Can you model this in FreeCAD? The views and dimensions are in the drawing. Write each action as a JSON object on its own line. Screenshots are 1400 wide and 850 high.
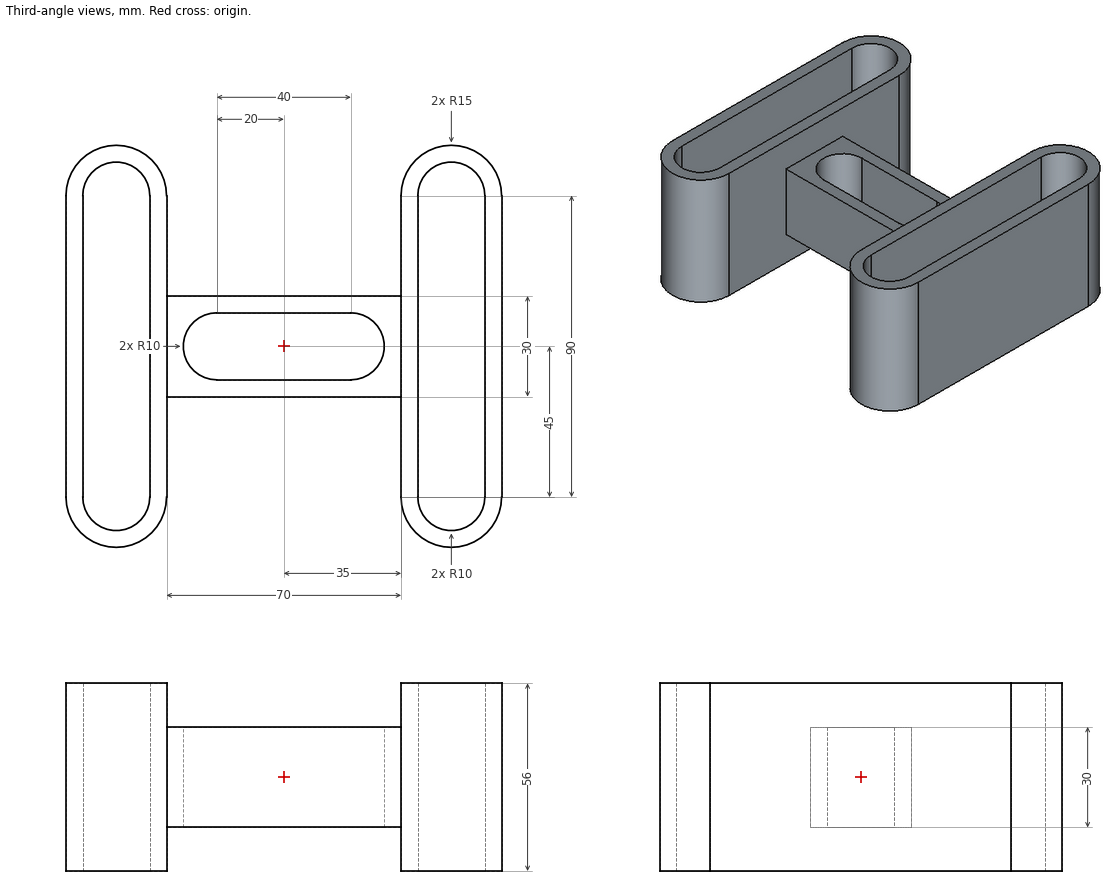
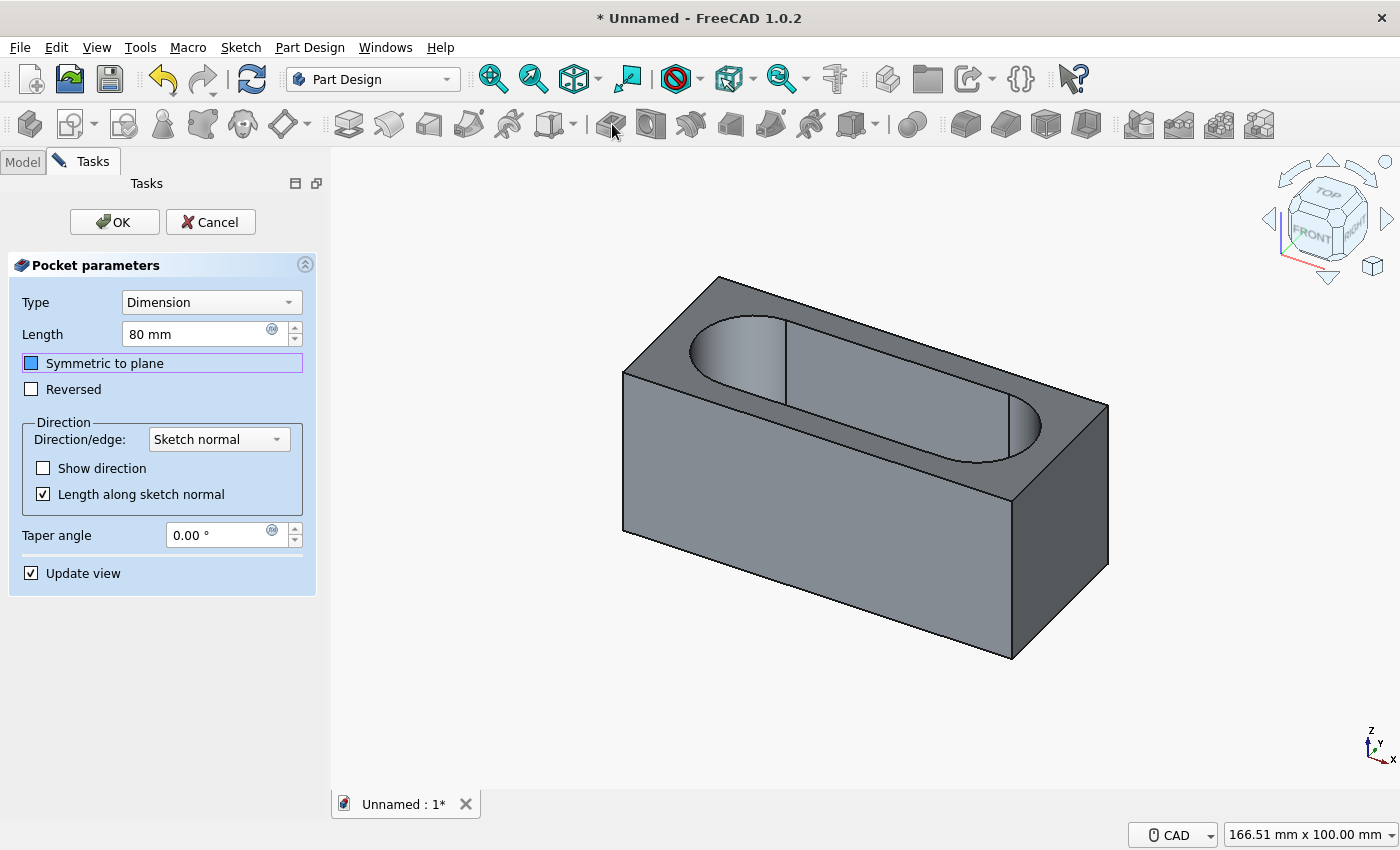
{"action": "left_click", "coordinate": [115, 222]}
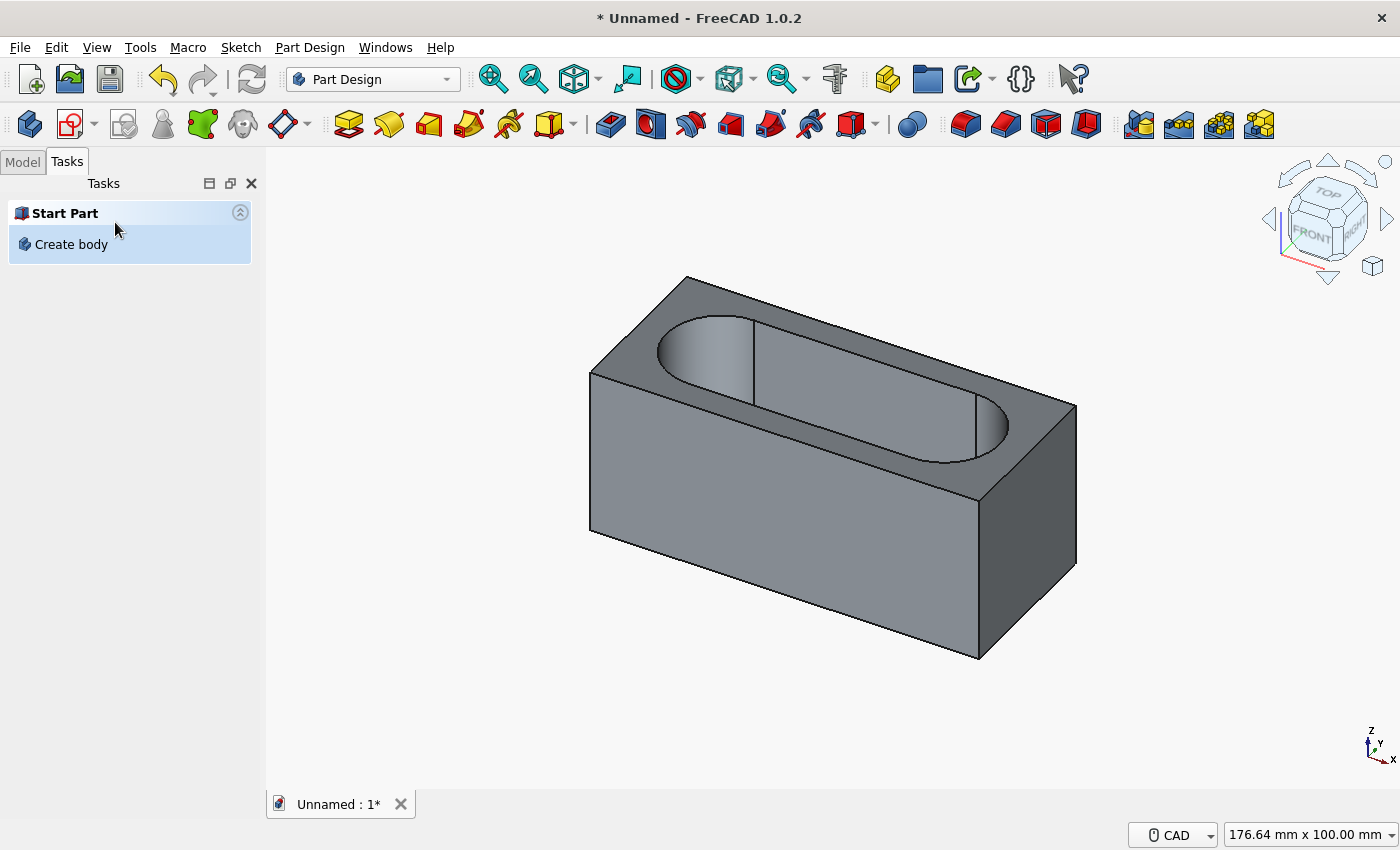
{"action": "left_click", "coordinate": [70, 124]}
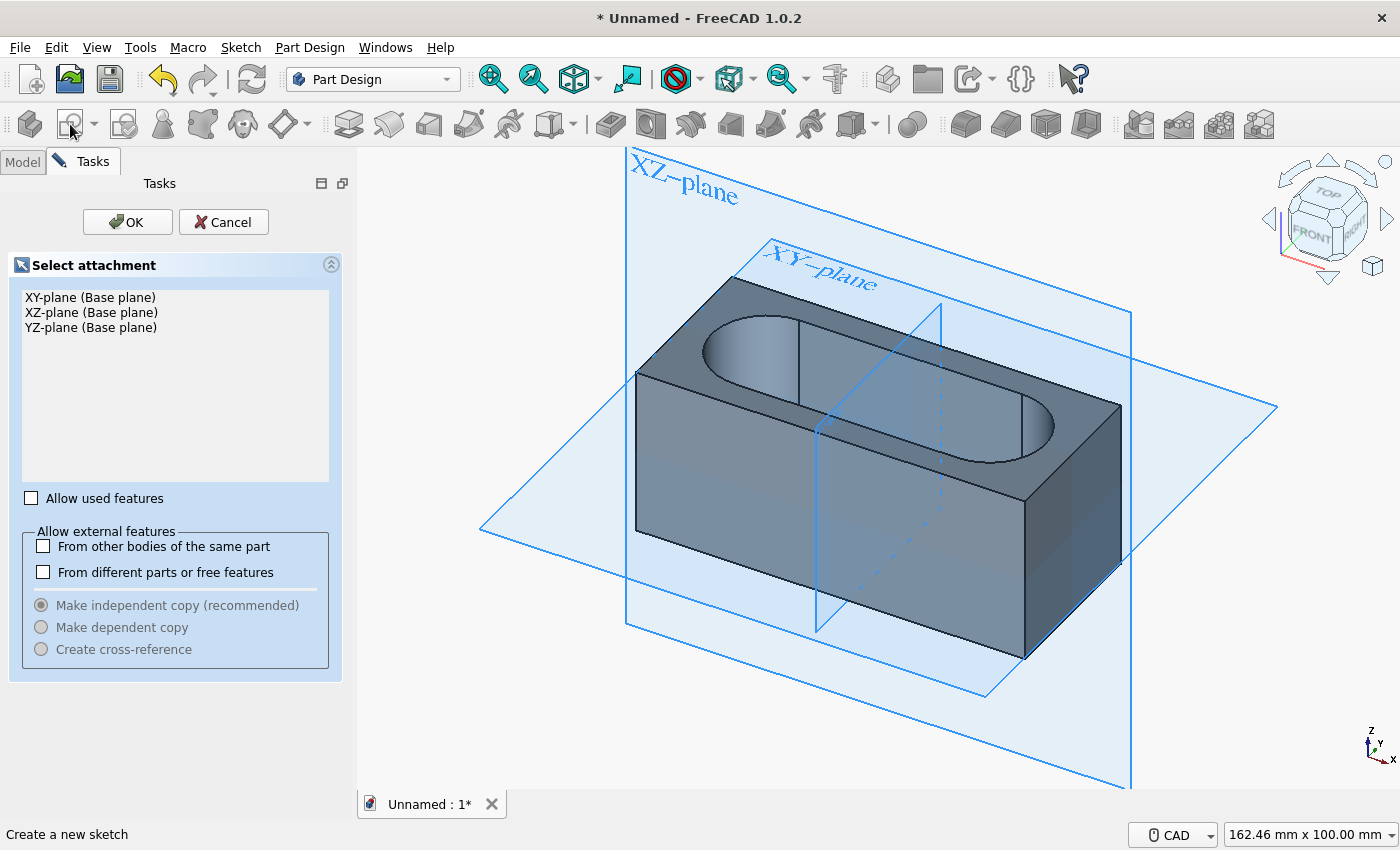
{"action": "left_click", "coordinate": [82, 298]}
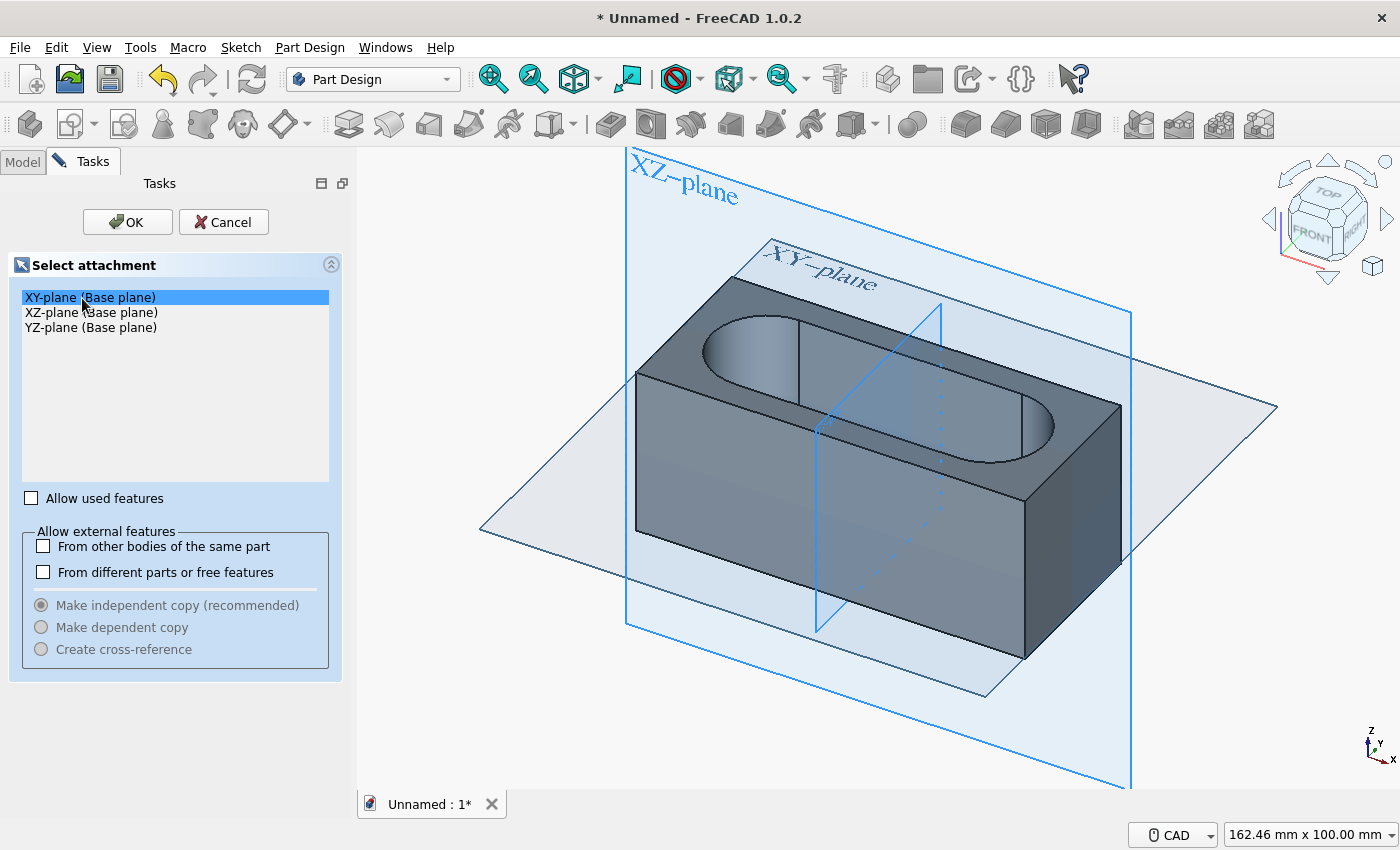
{"action": "left_click", "coordinate": [128, 222]}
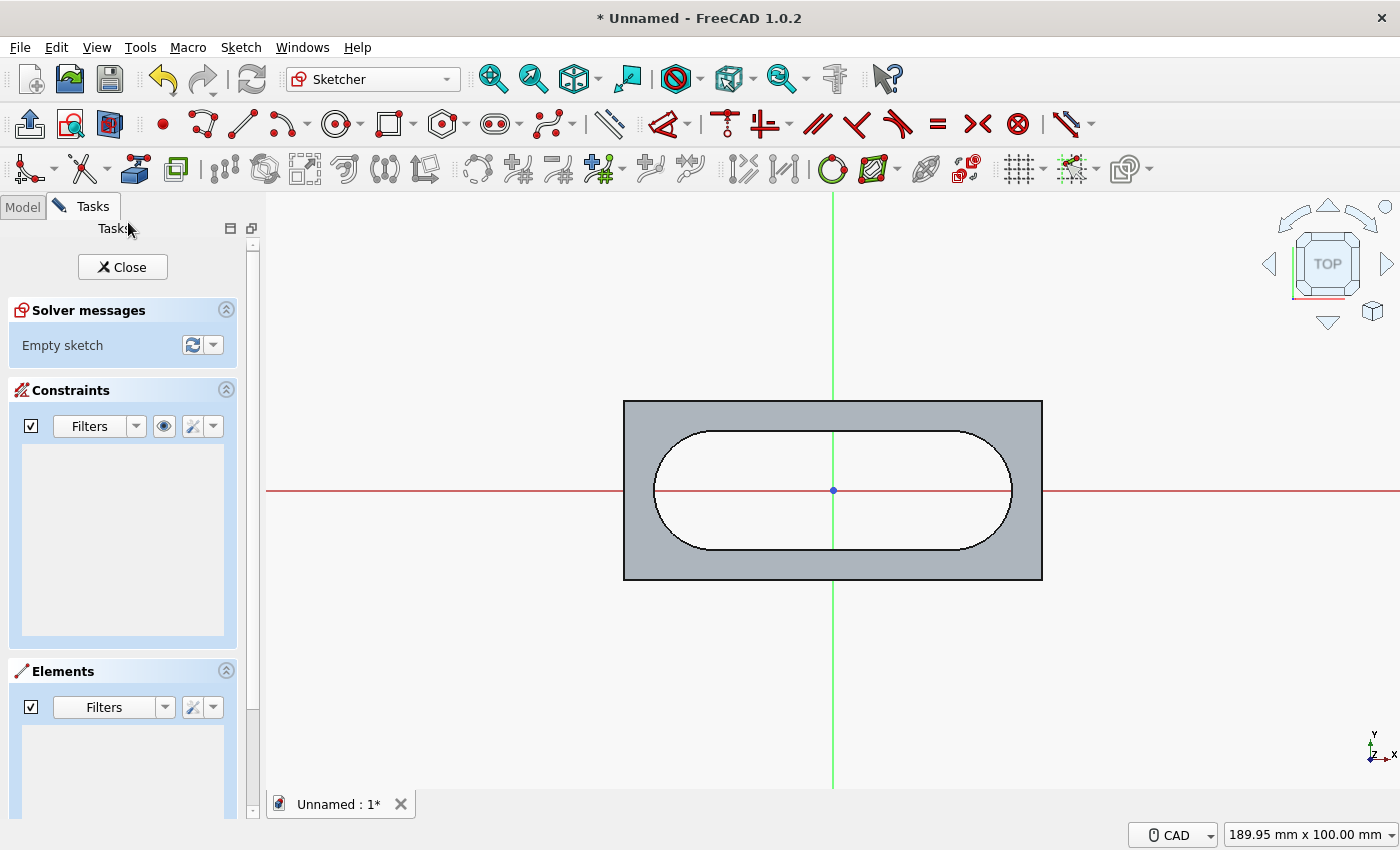
{"action": "key", "text": "q s"}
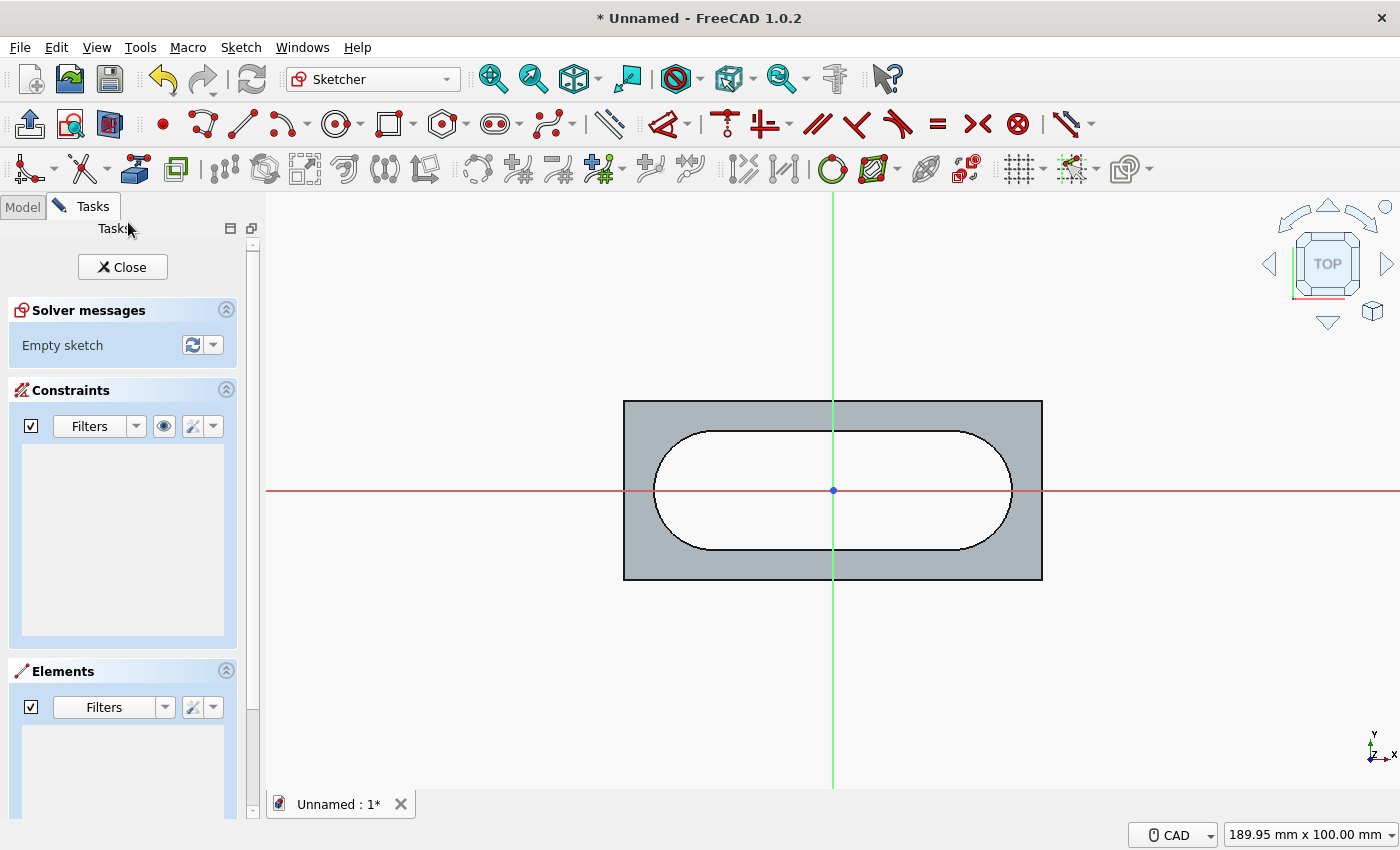
{"action": "scroll", "coordinate": [445, 491], "scroll_direction": "down", "scroll_amount": 3}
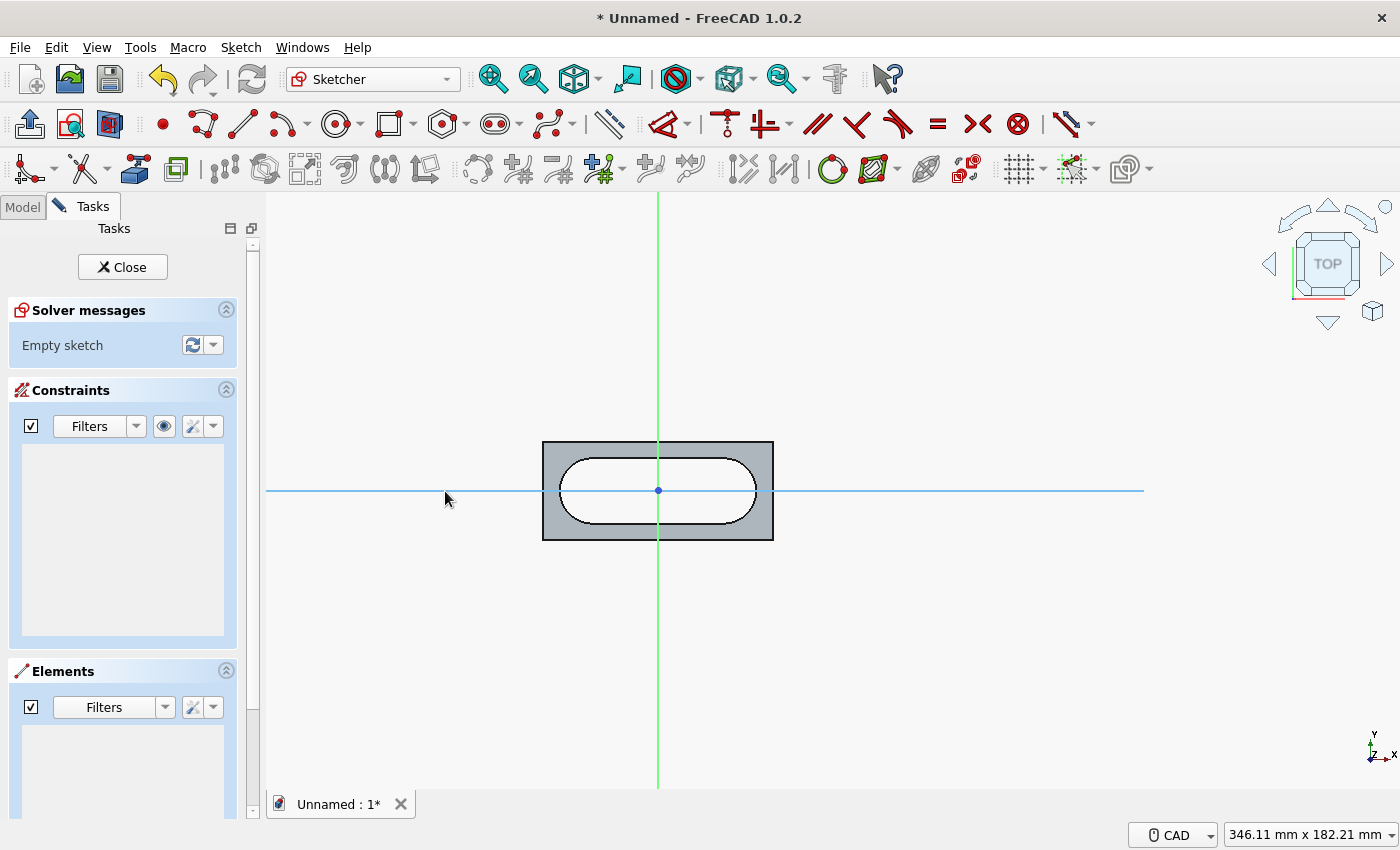
{"action": "left_click", "coordinate": [496, 124]}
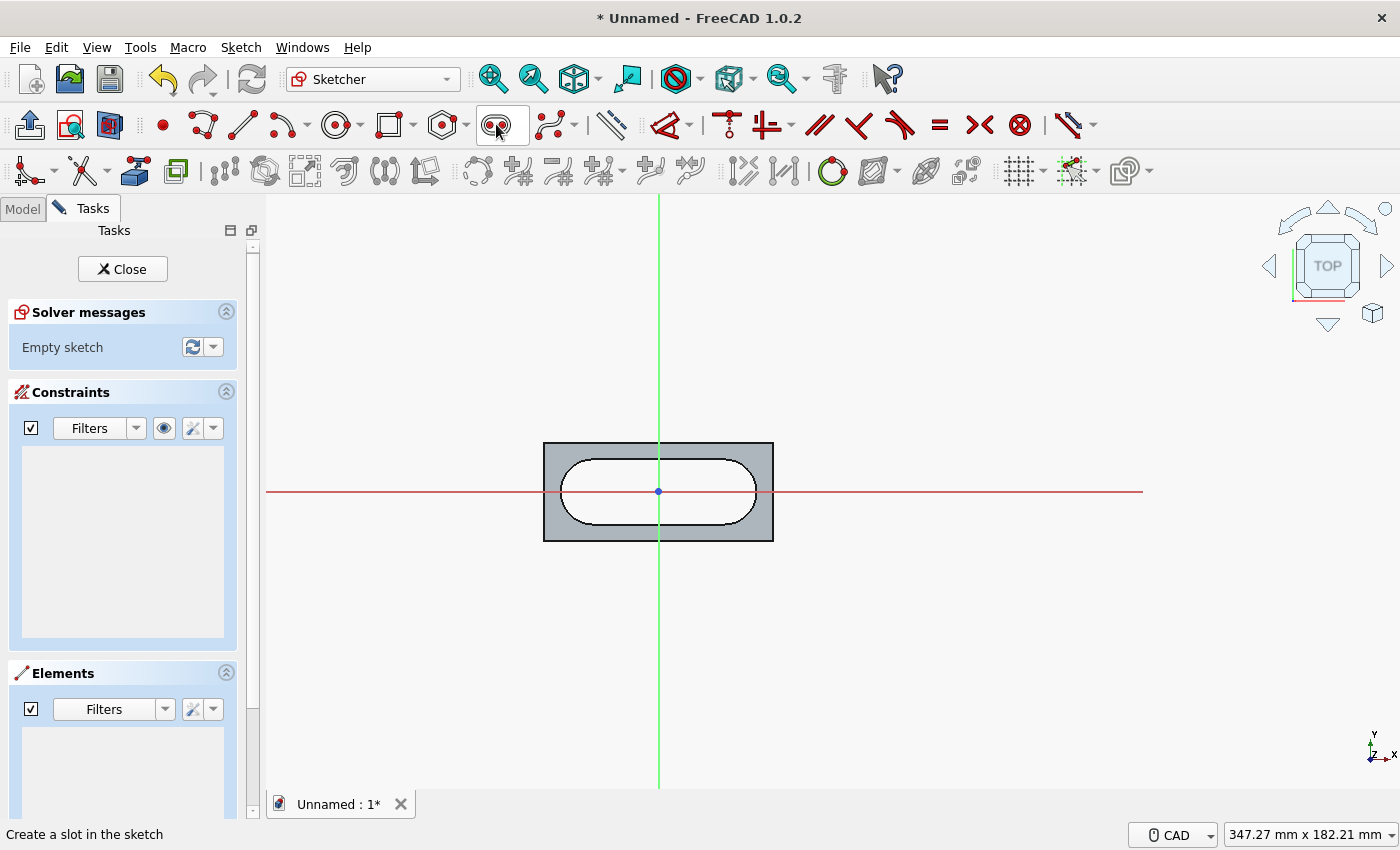
{"action": "left_click", "coordinate": [822, 639]}